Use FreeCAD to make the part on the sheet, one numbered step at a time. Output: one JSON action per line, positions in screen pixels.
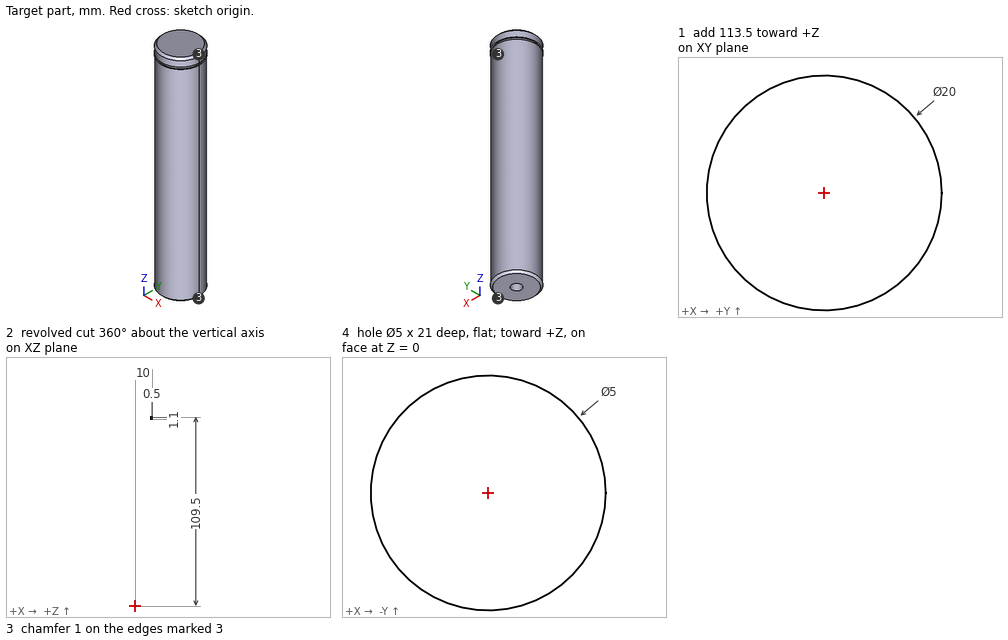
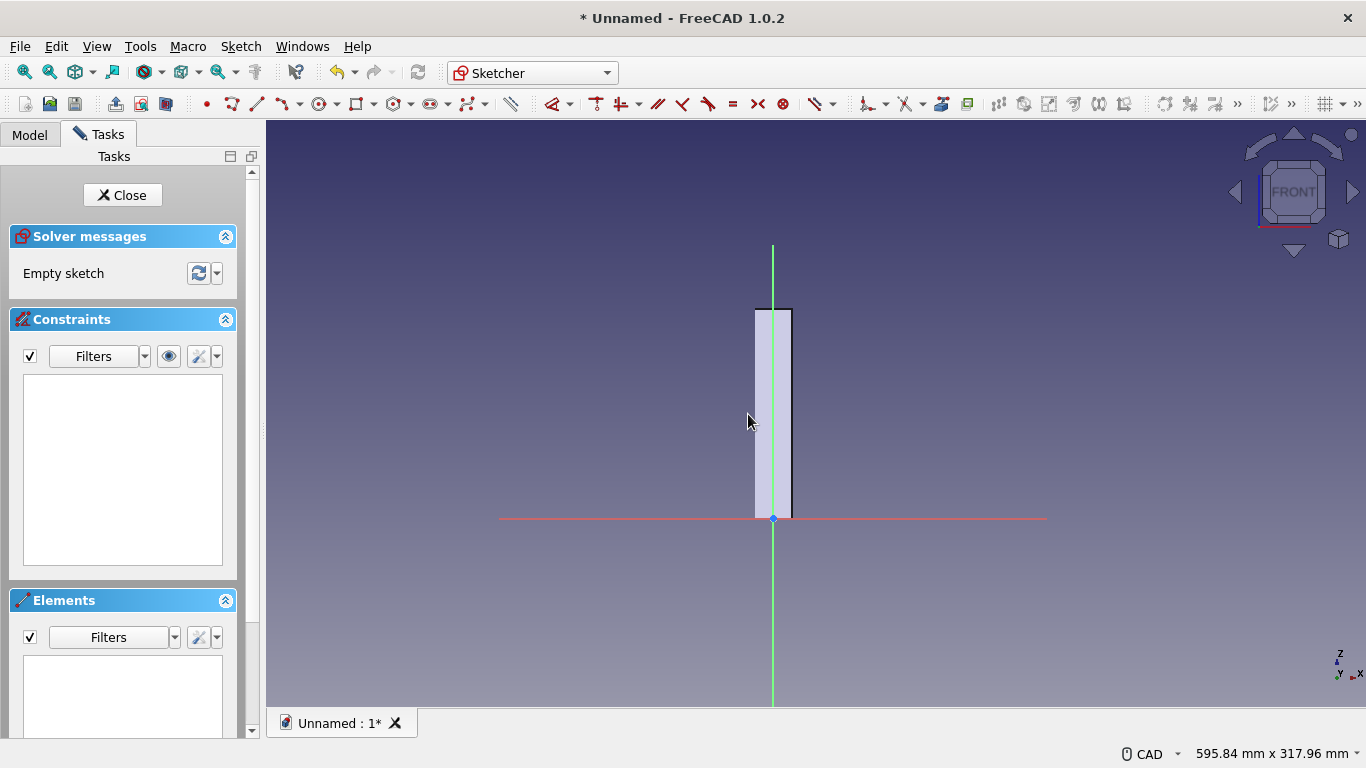
{"action": "scroll", "coordinate": [794, 313], "scroll_direction": "up", "scroll_amount": 15}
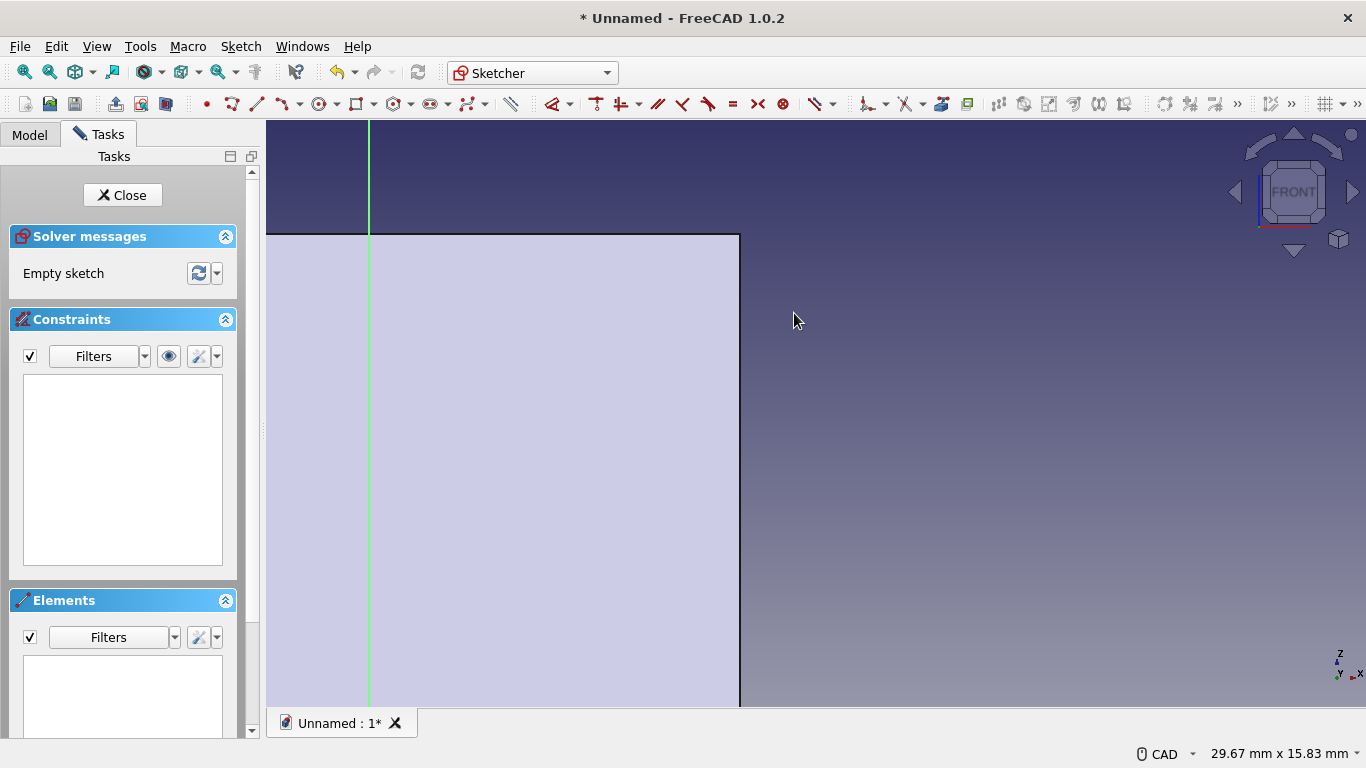
{"action": "scroll", "coordinate": [728, 401], "scroll_direction": "up", "scroll_amount": 11}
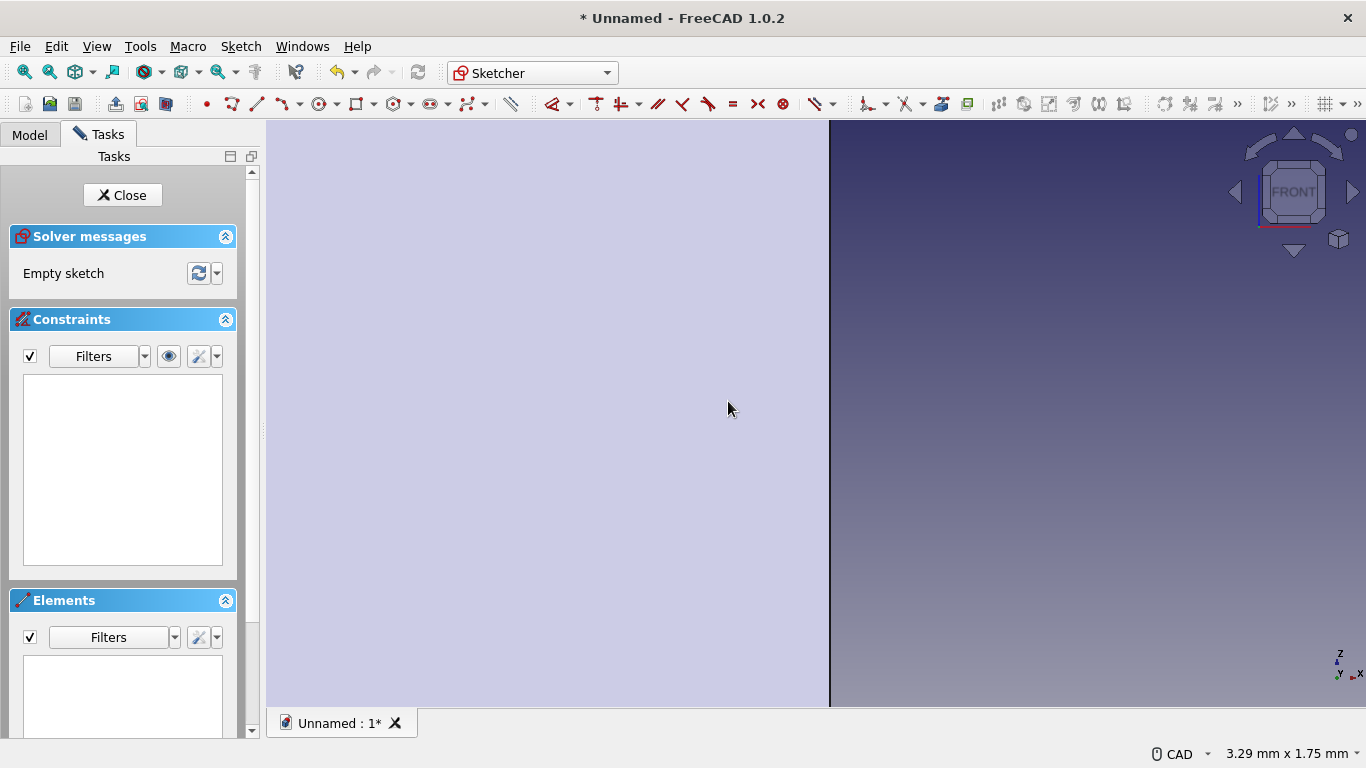
{"action": "key", "text": "g r"}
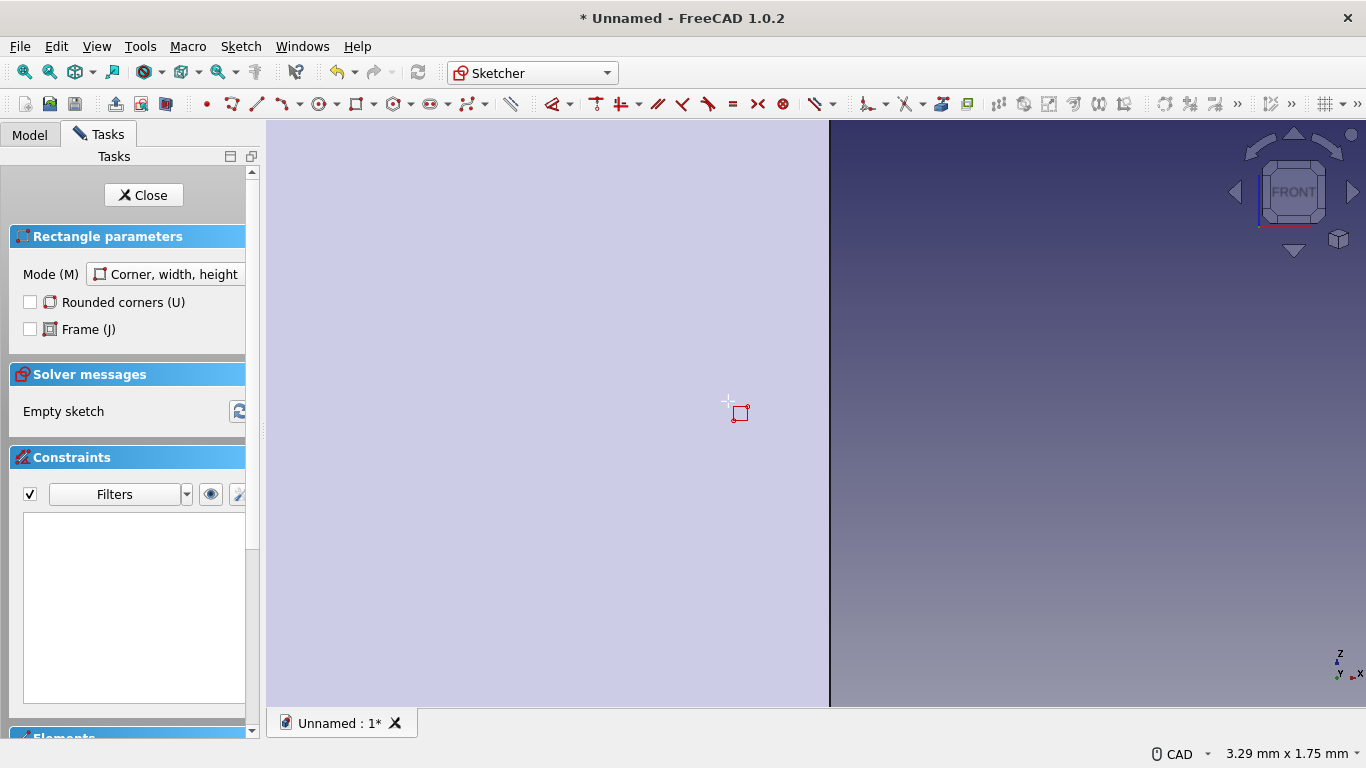
{"action": "left_click", "coordinate": [663, 226]}
{"action": "left_click", "coordinate": [830, 594]}
{"action": "key", "text": "Escape"}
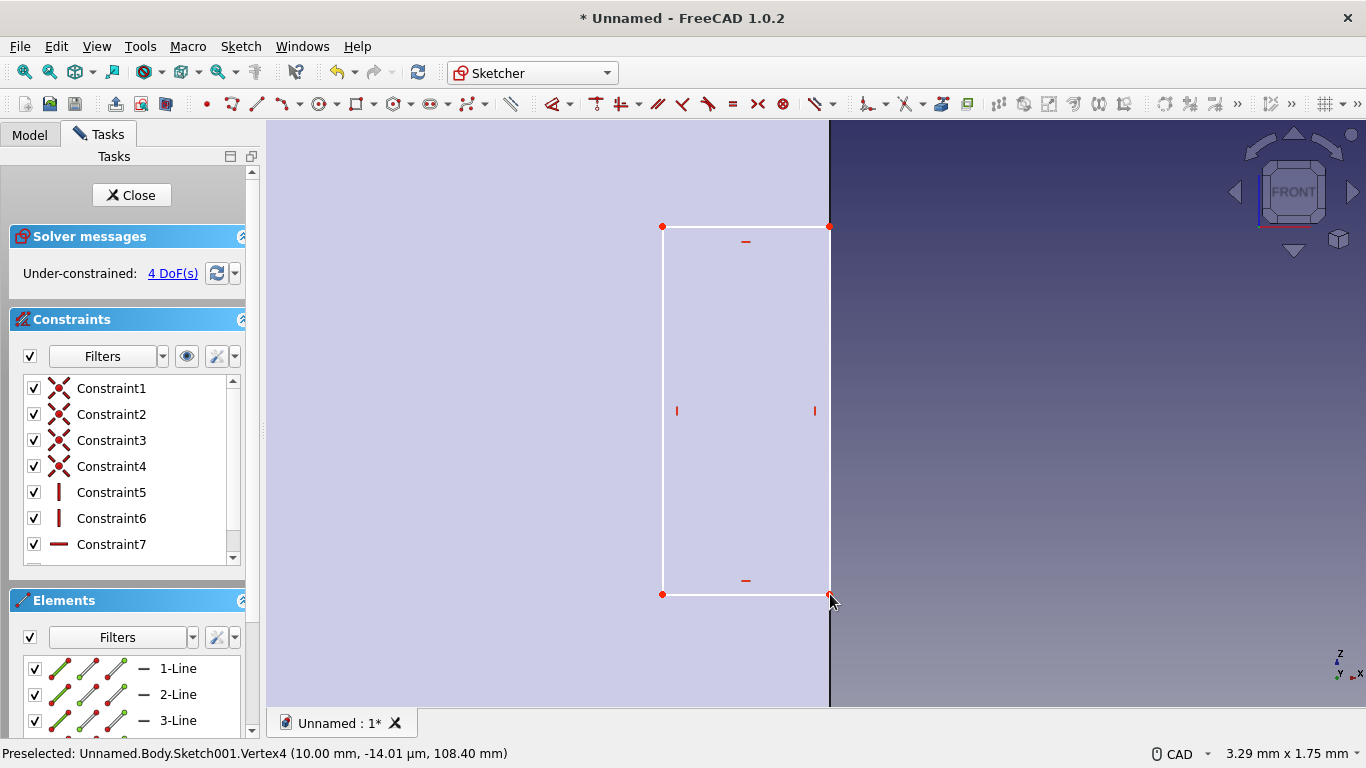
{"action": "key", "text": "d"}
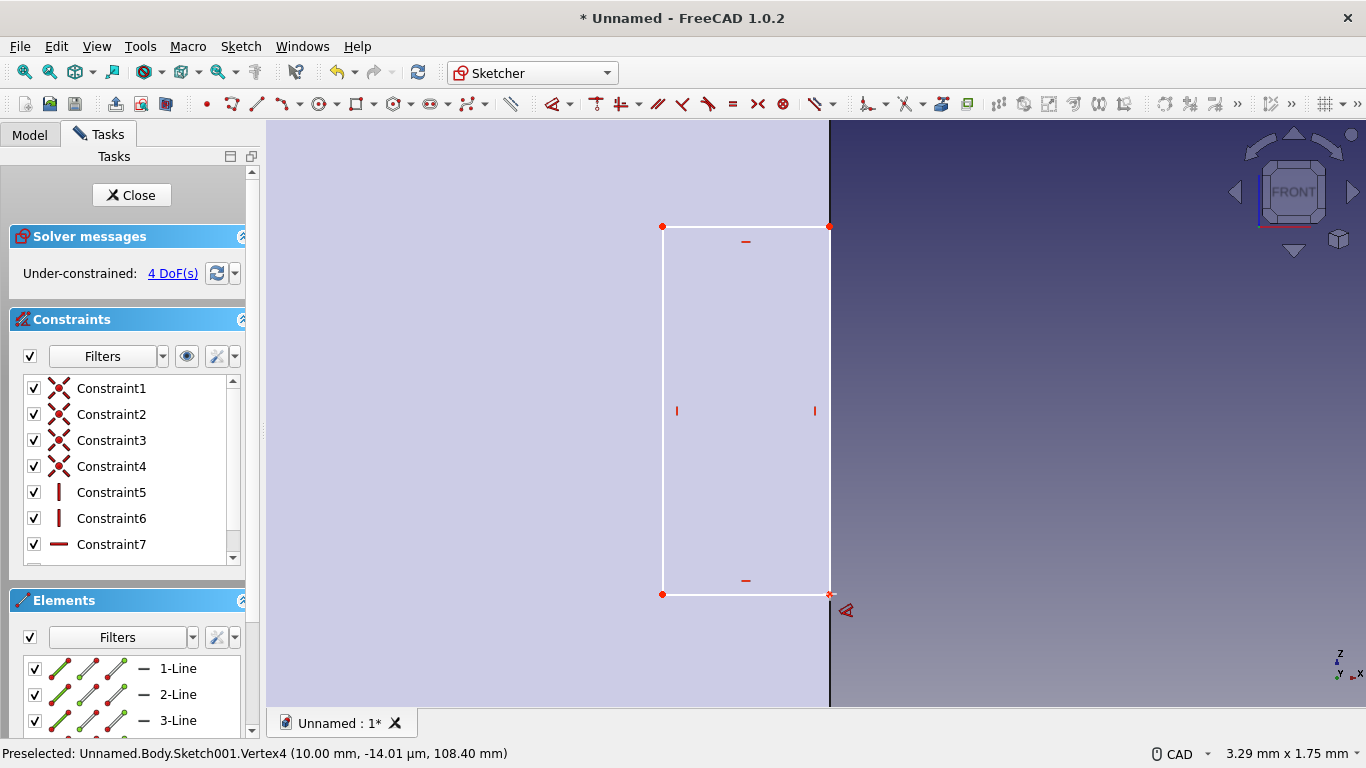
{"action": "left_click", "coordinate": [663, 337]}
{"action": "left_click", "coordinate": [629, 411]}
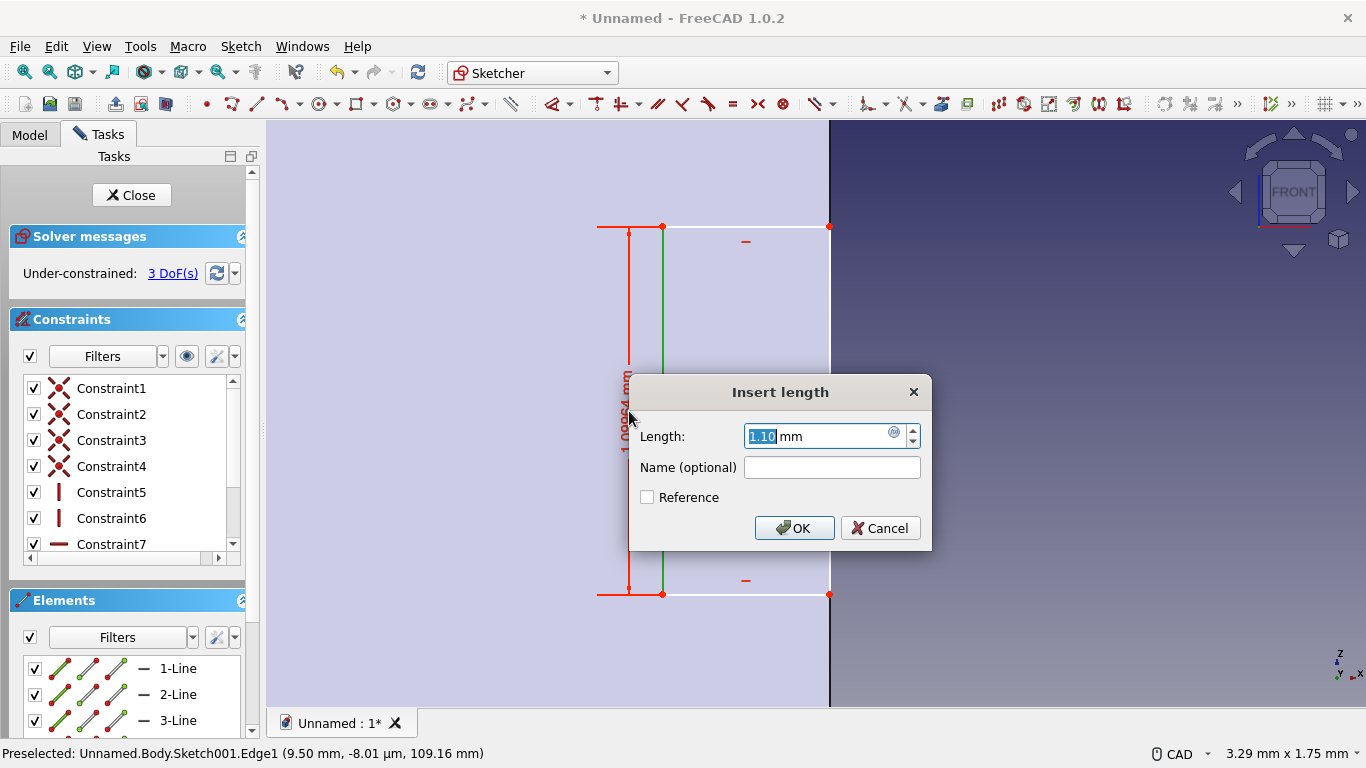
{"action": "type", "text": "1.1"}
{"action": "key", "text": "Return"}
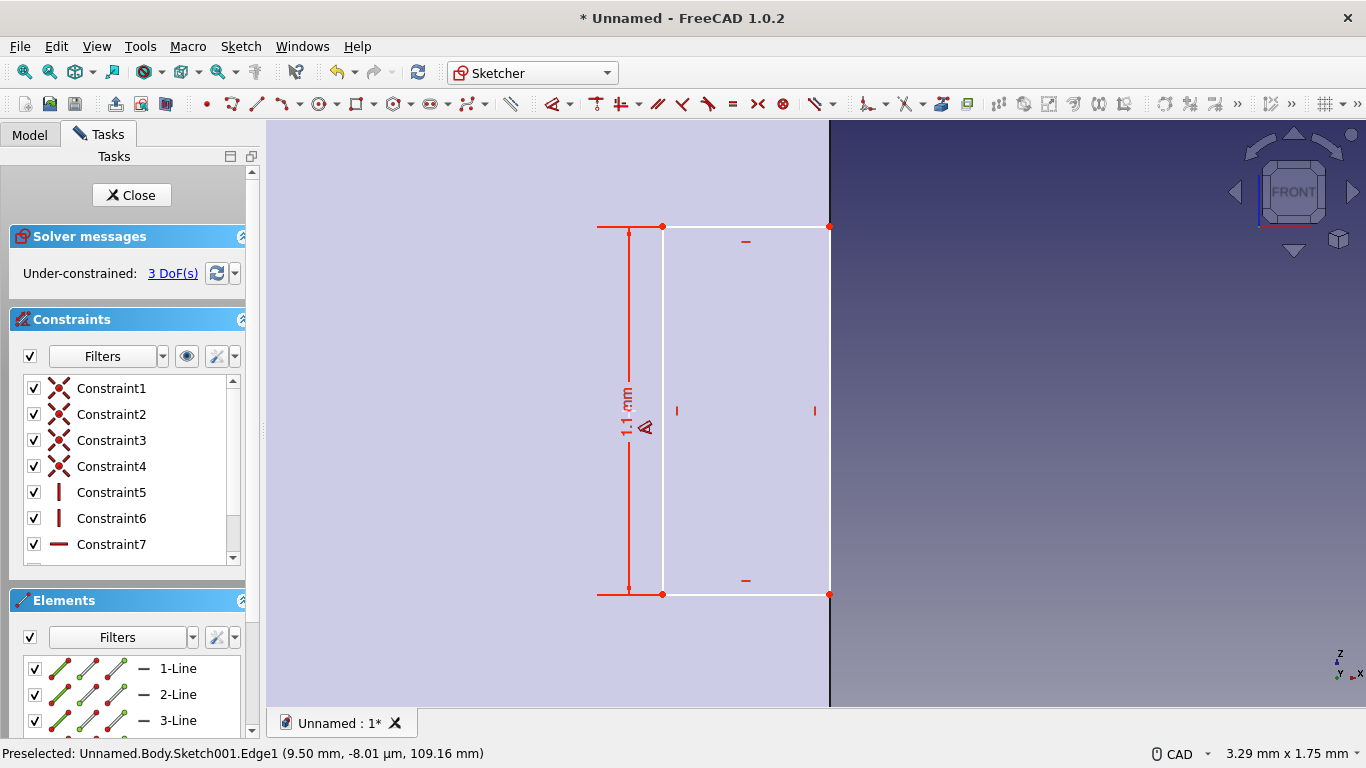
{"action": "left_click", "coordinate": [713, 595]}
{"action": "left_click", "coordinate": [746, 629]}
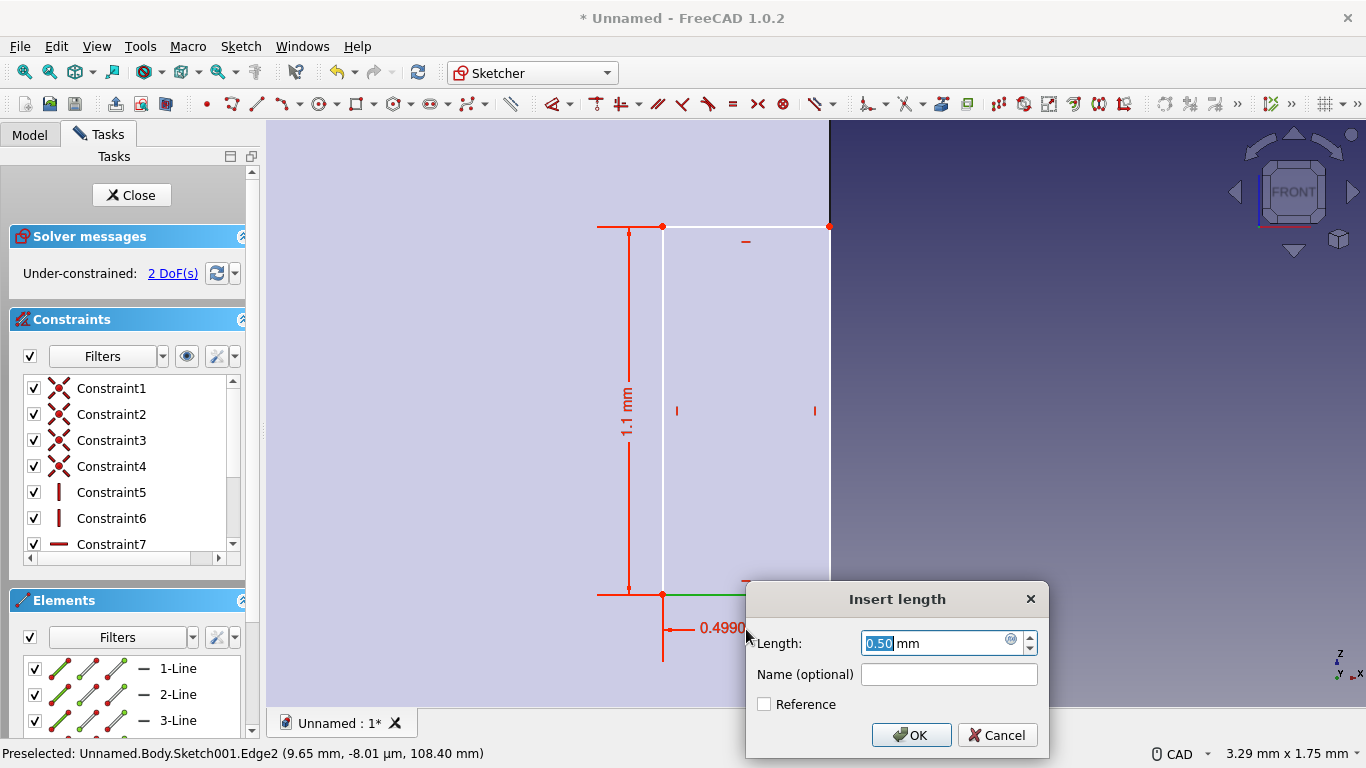
{"action": "type", "text": "0.5"}
{"action": "key", "text": "Return"}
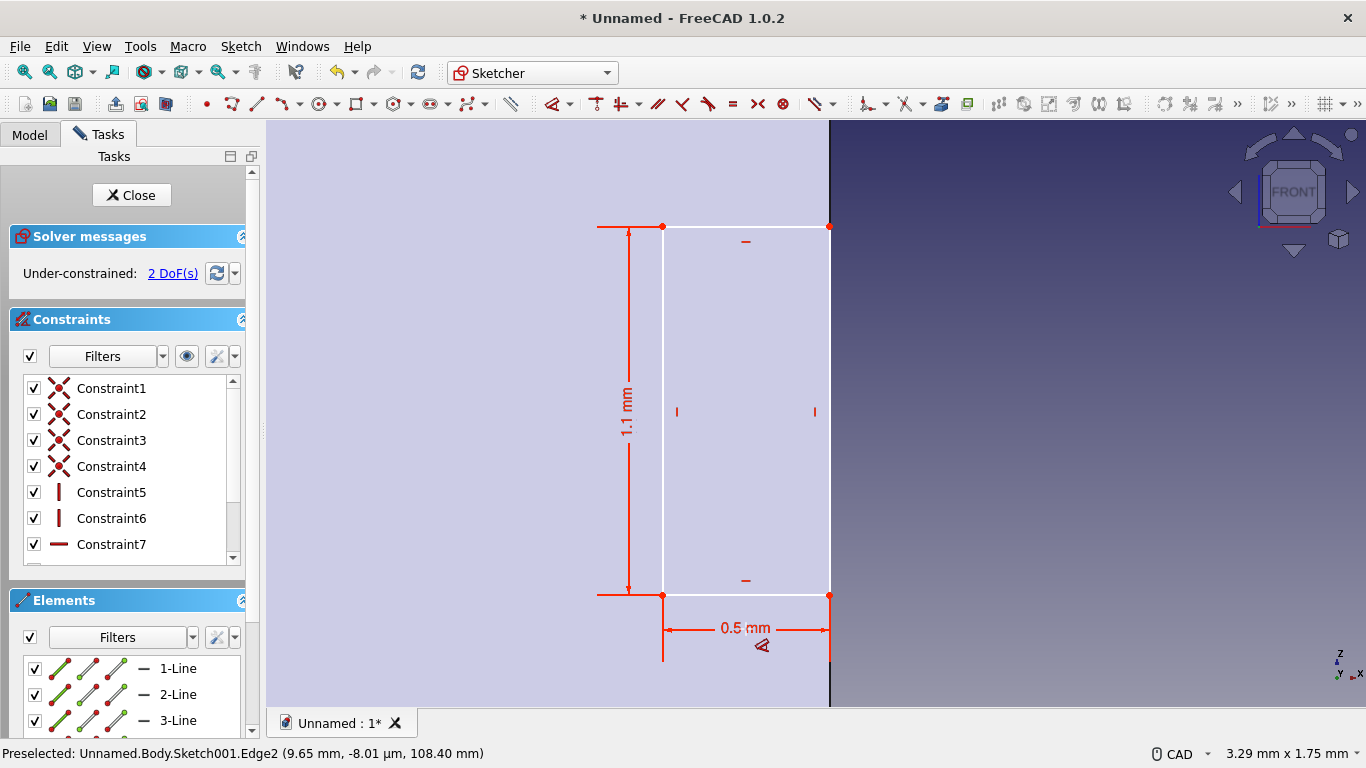
{"action": "left_click", "coordinate": [830, 595]}
{"action": "left_click", "coordinate": [562, 561]}